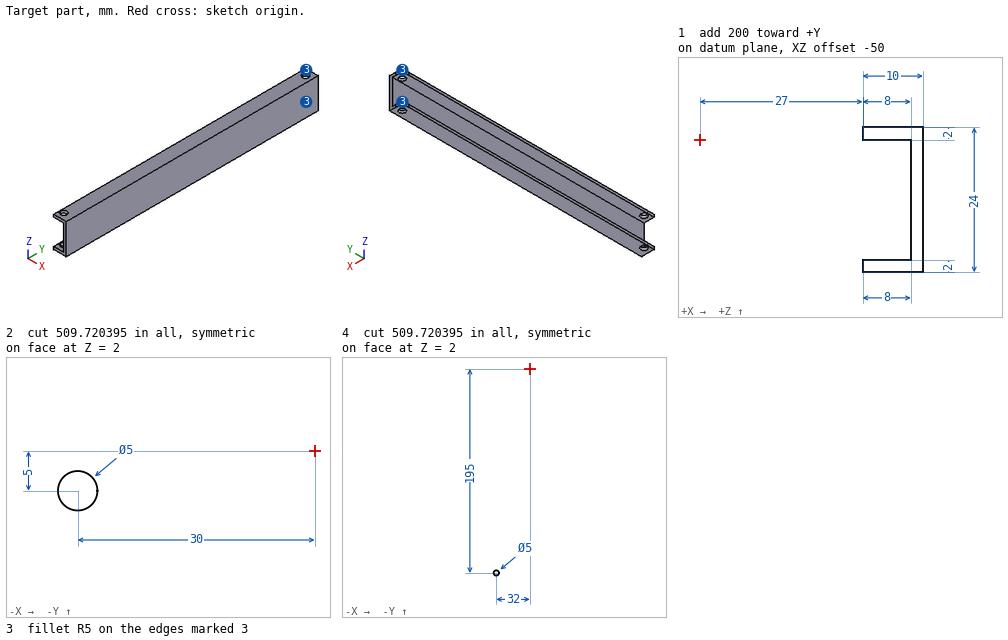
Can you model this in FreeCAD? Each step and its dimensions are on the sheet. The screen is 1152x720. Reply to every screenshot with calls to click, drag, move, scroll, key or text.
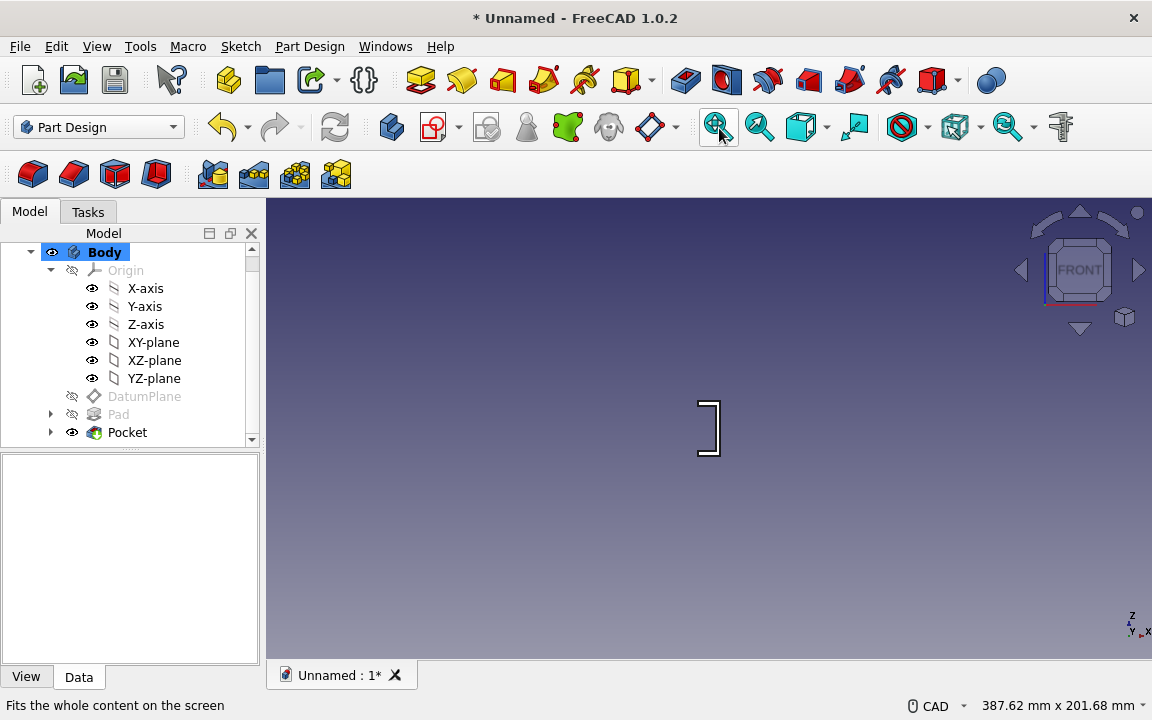
key(3)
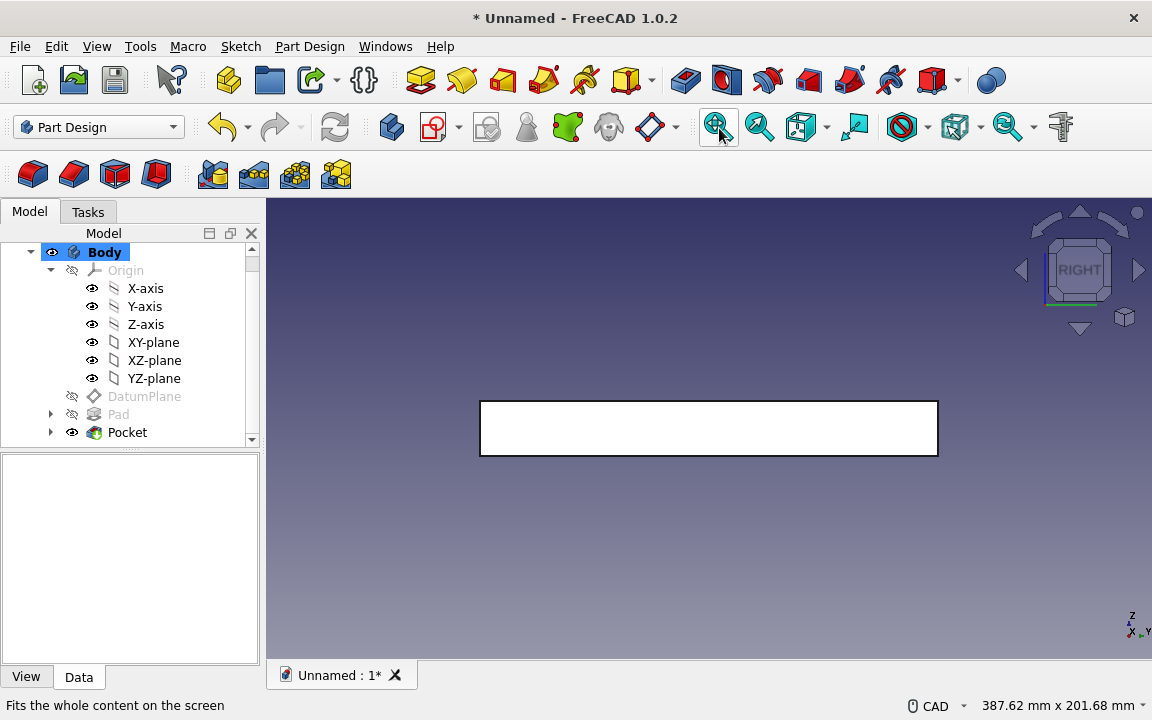
scroll(938, 402, up, 11)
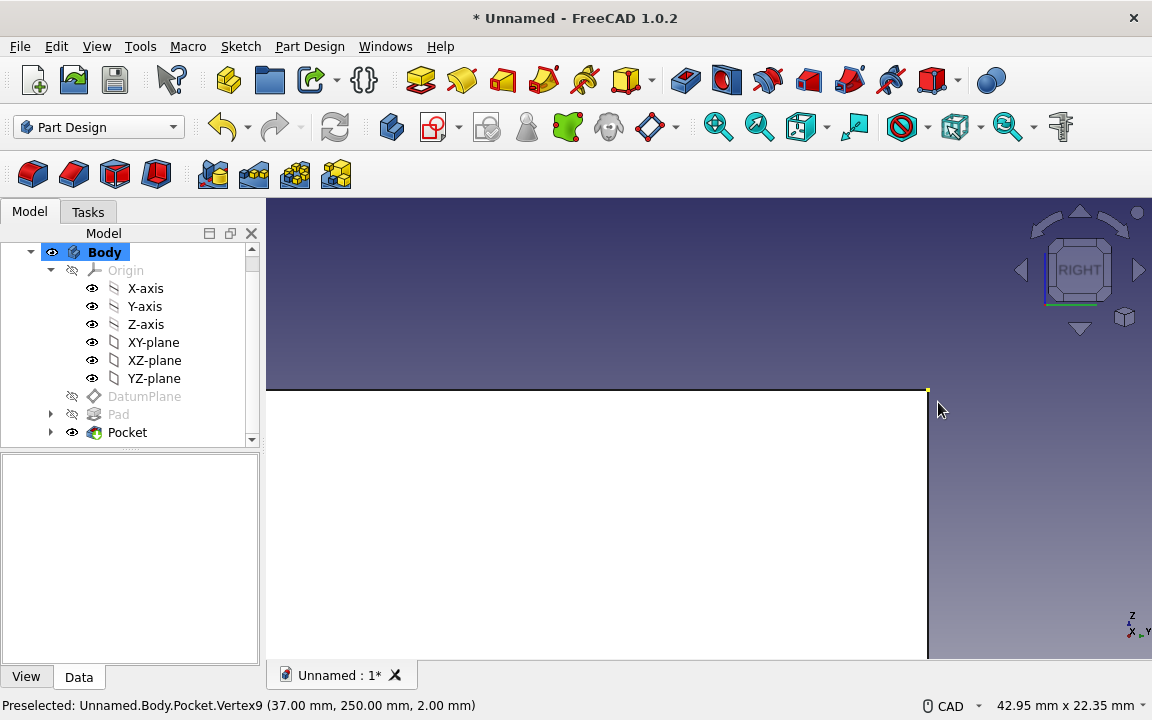
click(719, 128)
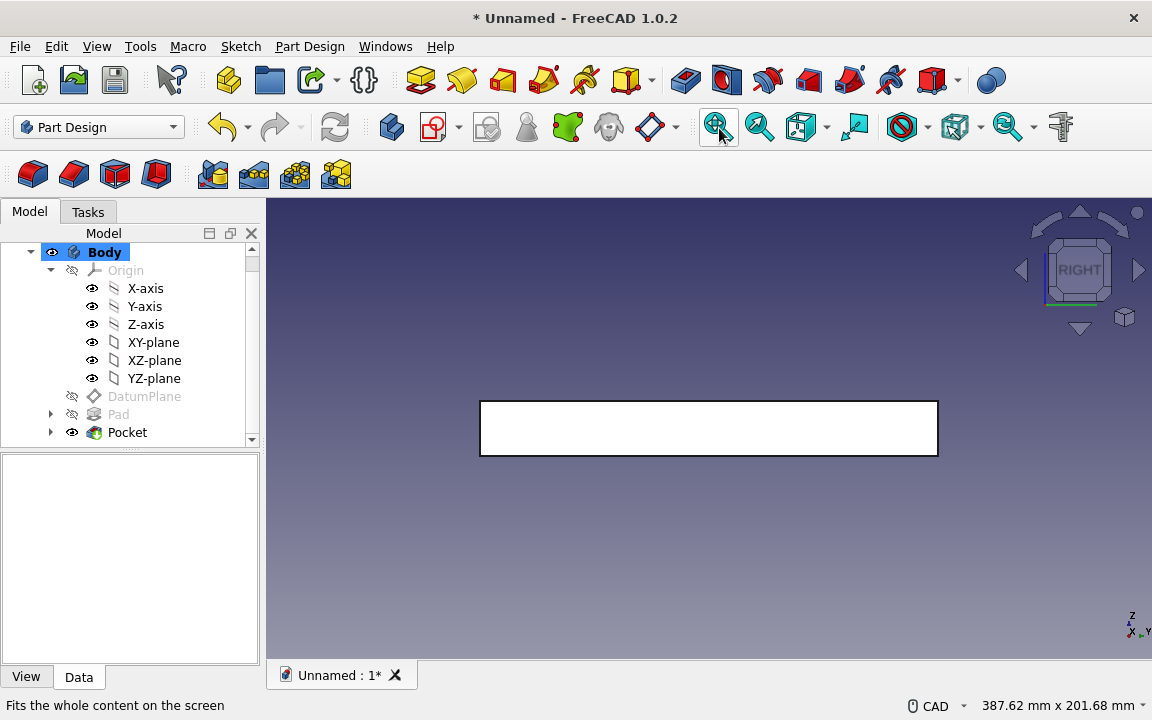
key(5)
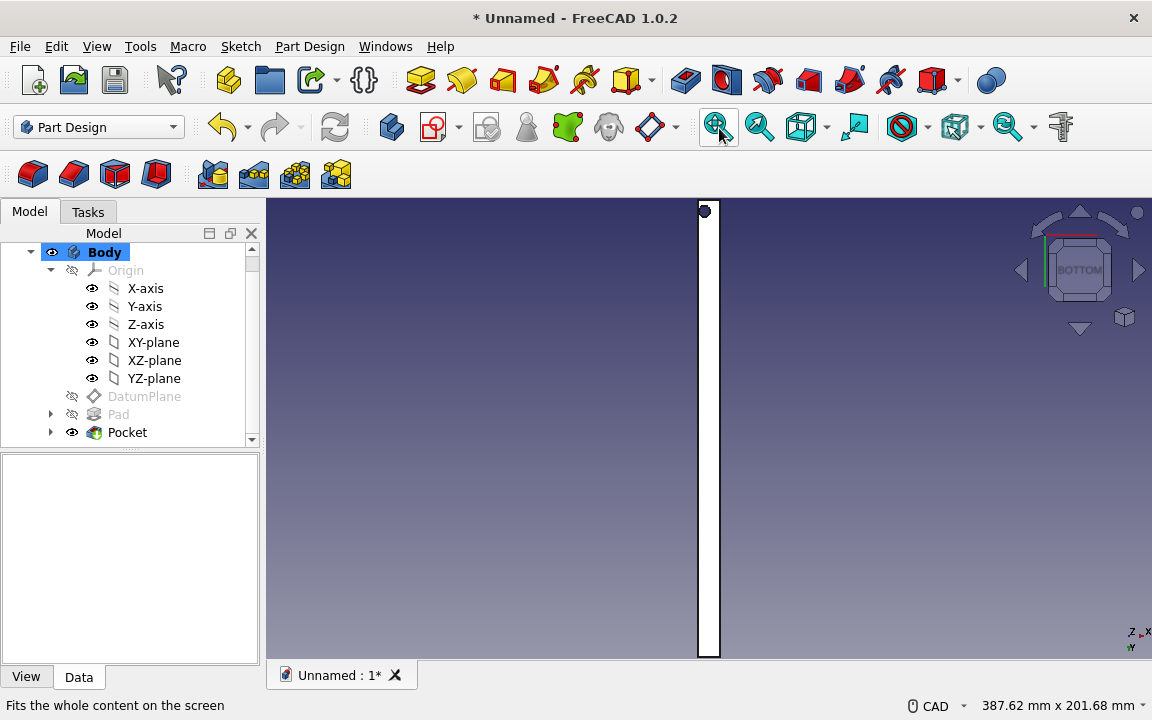
key(4)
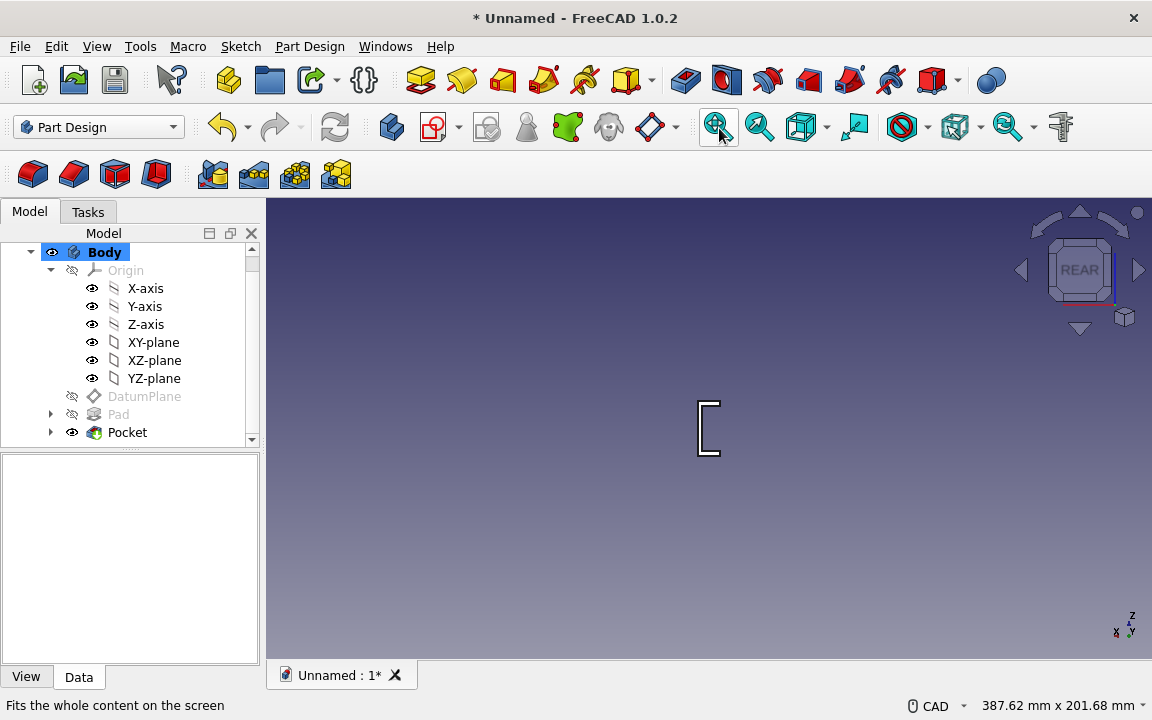
click(719, 128)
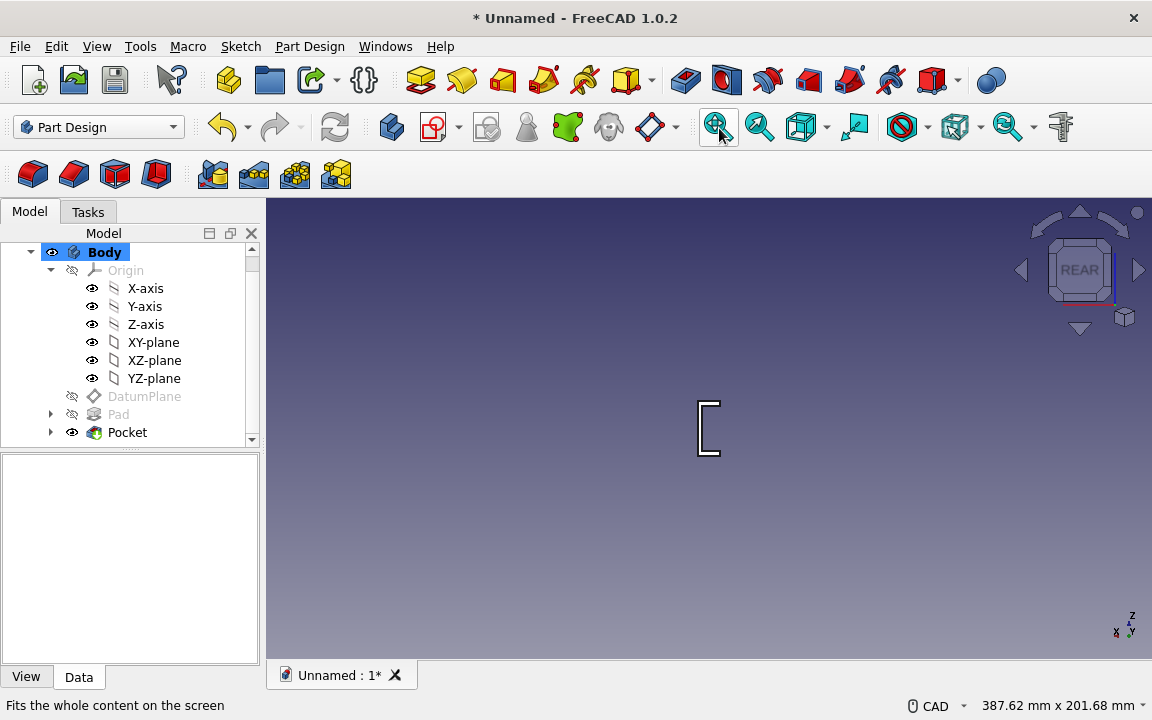
scroll(720, 402, up, 11)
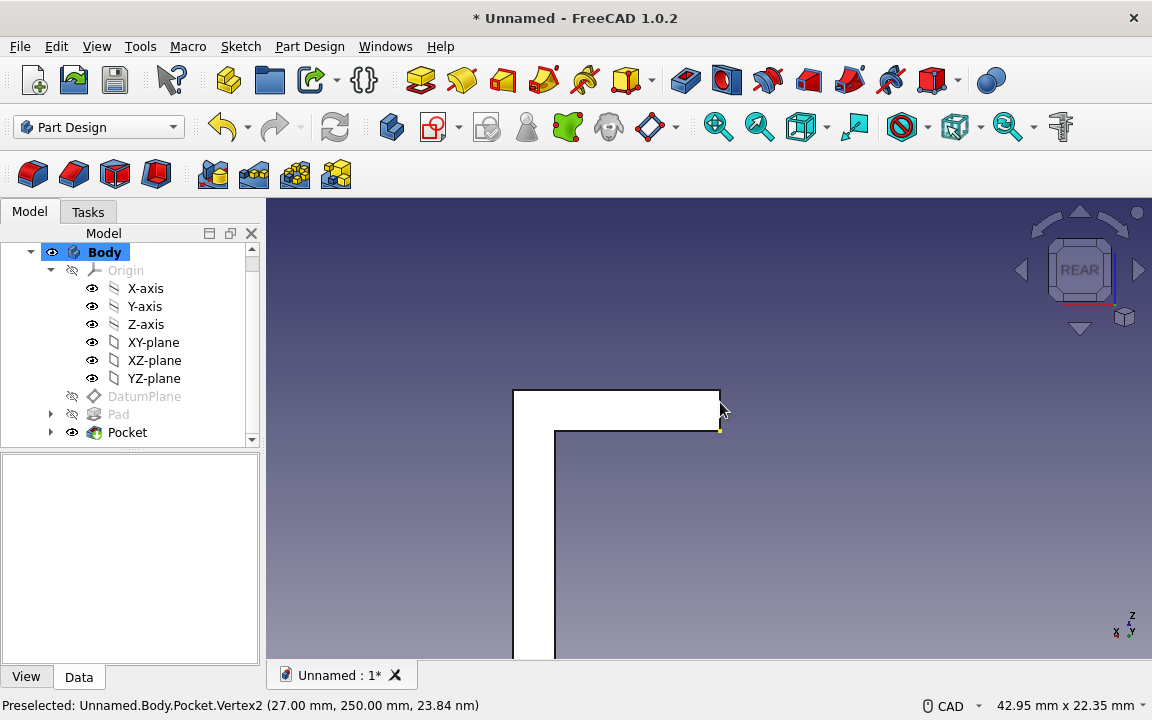
click(720, 410)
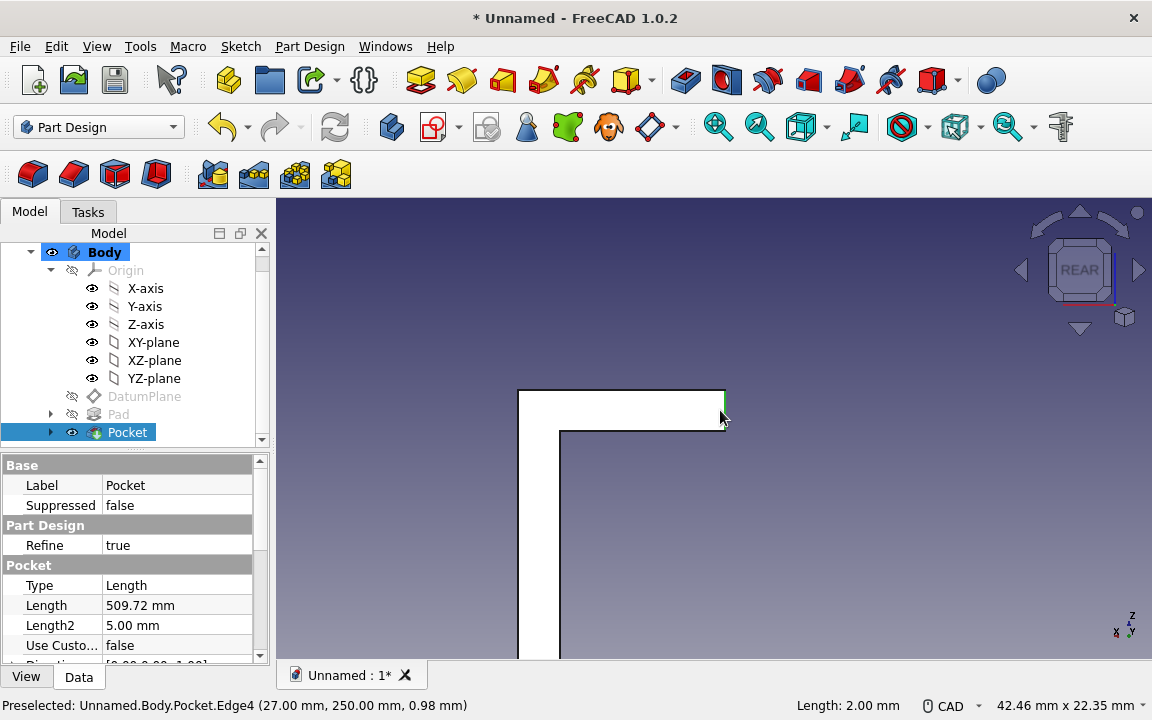
click(719, 128)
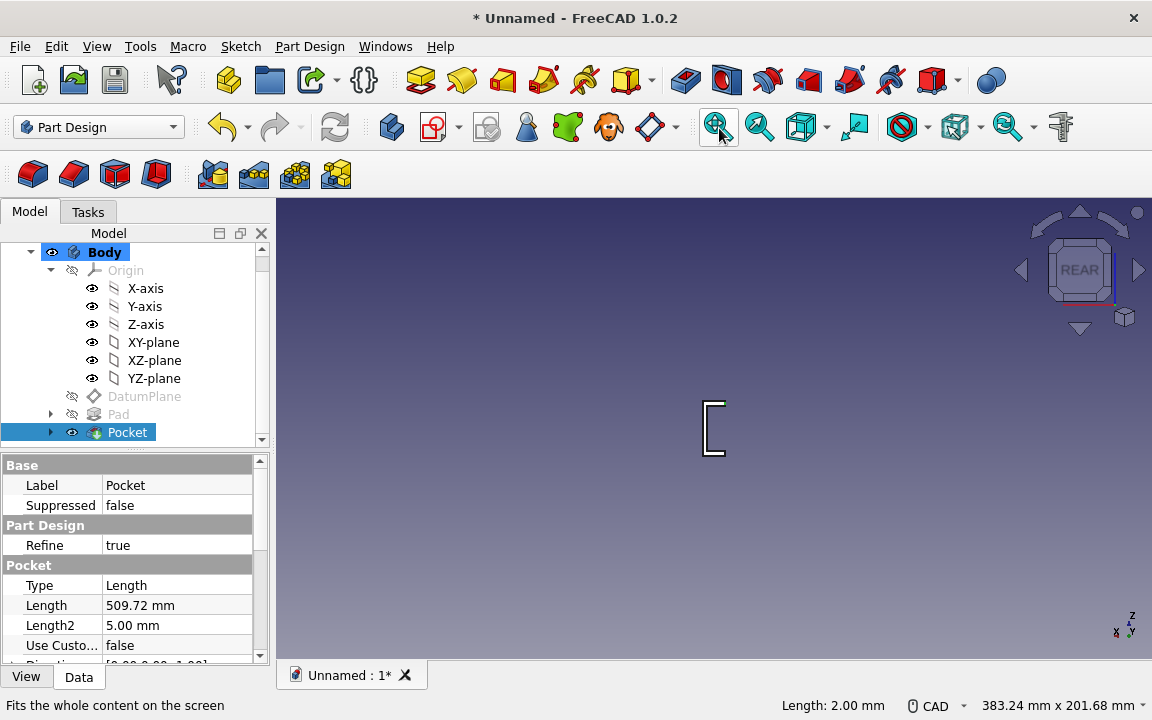
key(6)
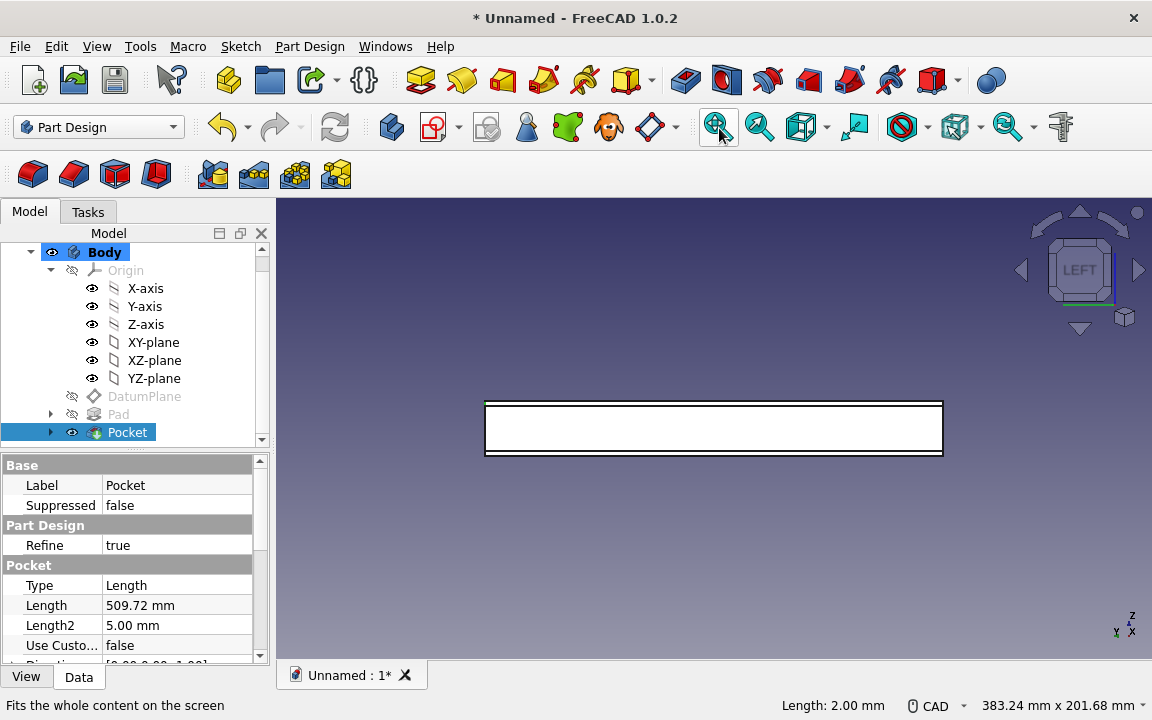
scroll(485, 453, up, 11)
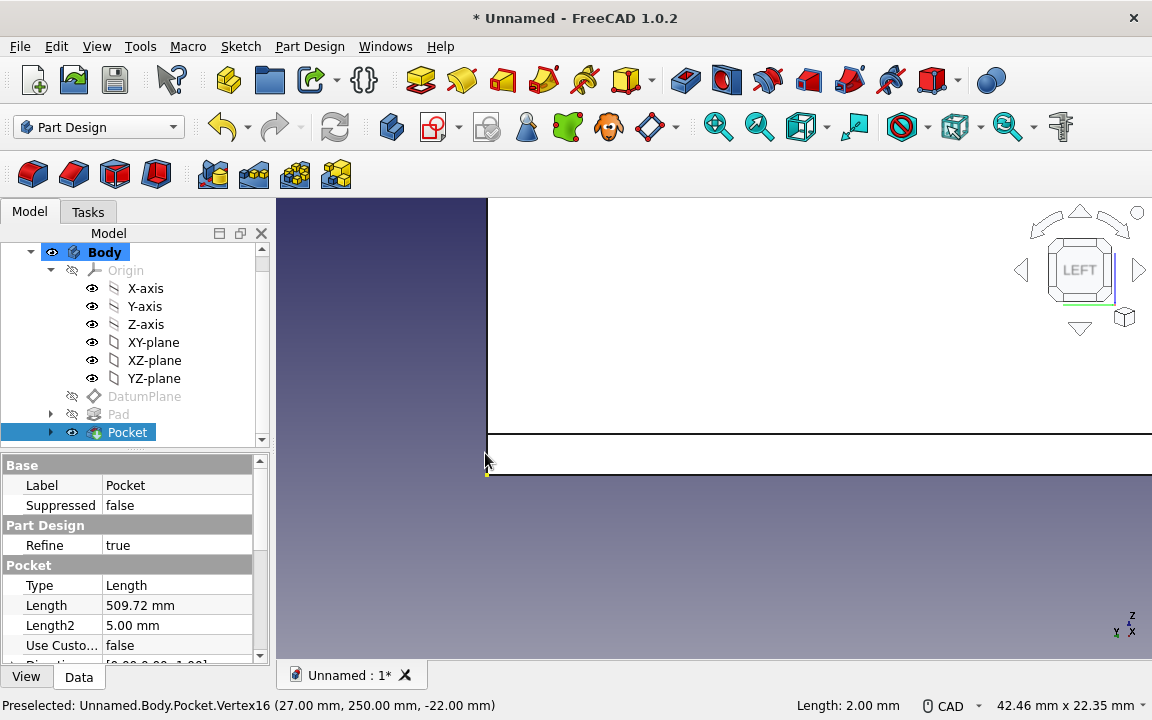
click(487, 453, ctrl)